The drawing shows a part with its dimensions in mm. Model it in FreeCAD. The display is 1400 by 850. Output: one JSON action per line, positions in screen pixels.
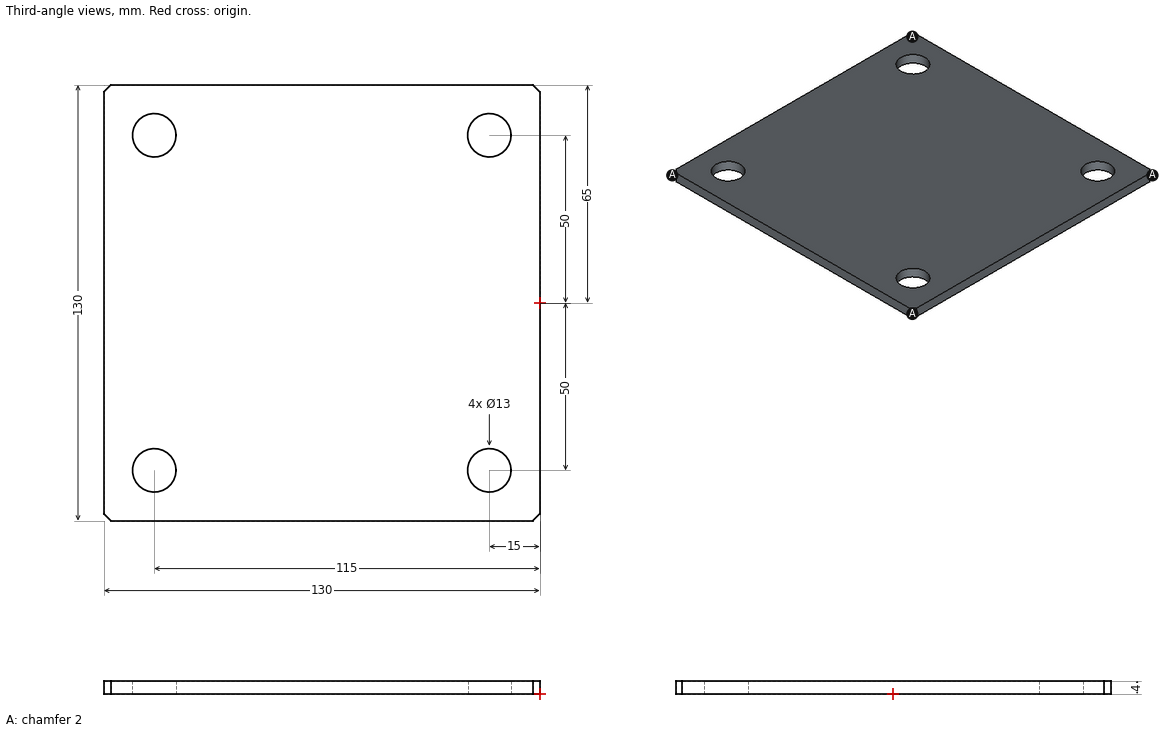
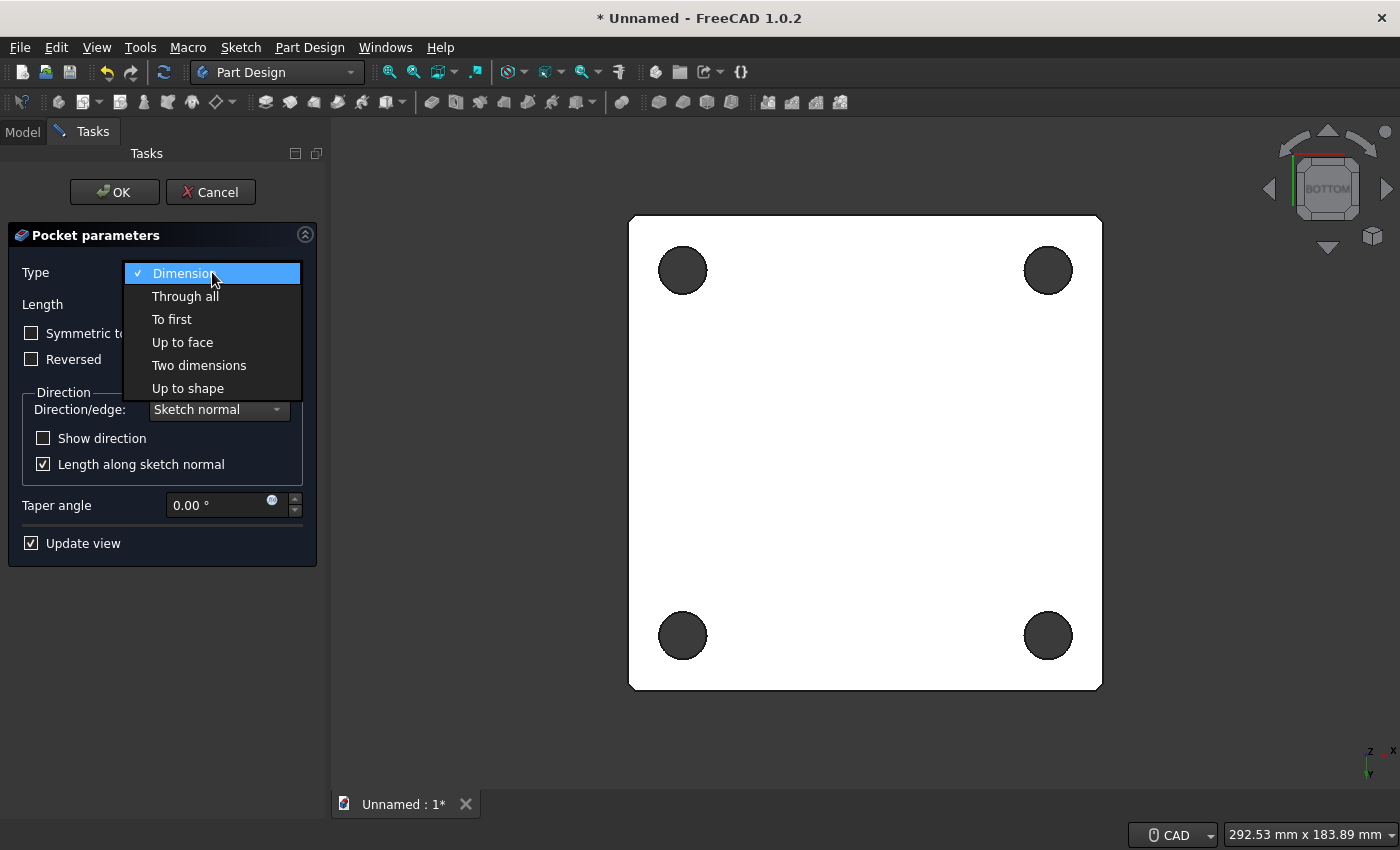
{"action": "left_click", "coordinate": [212, 296]}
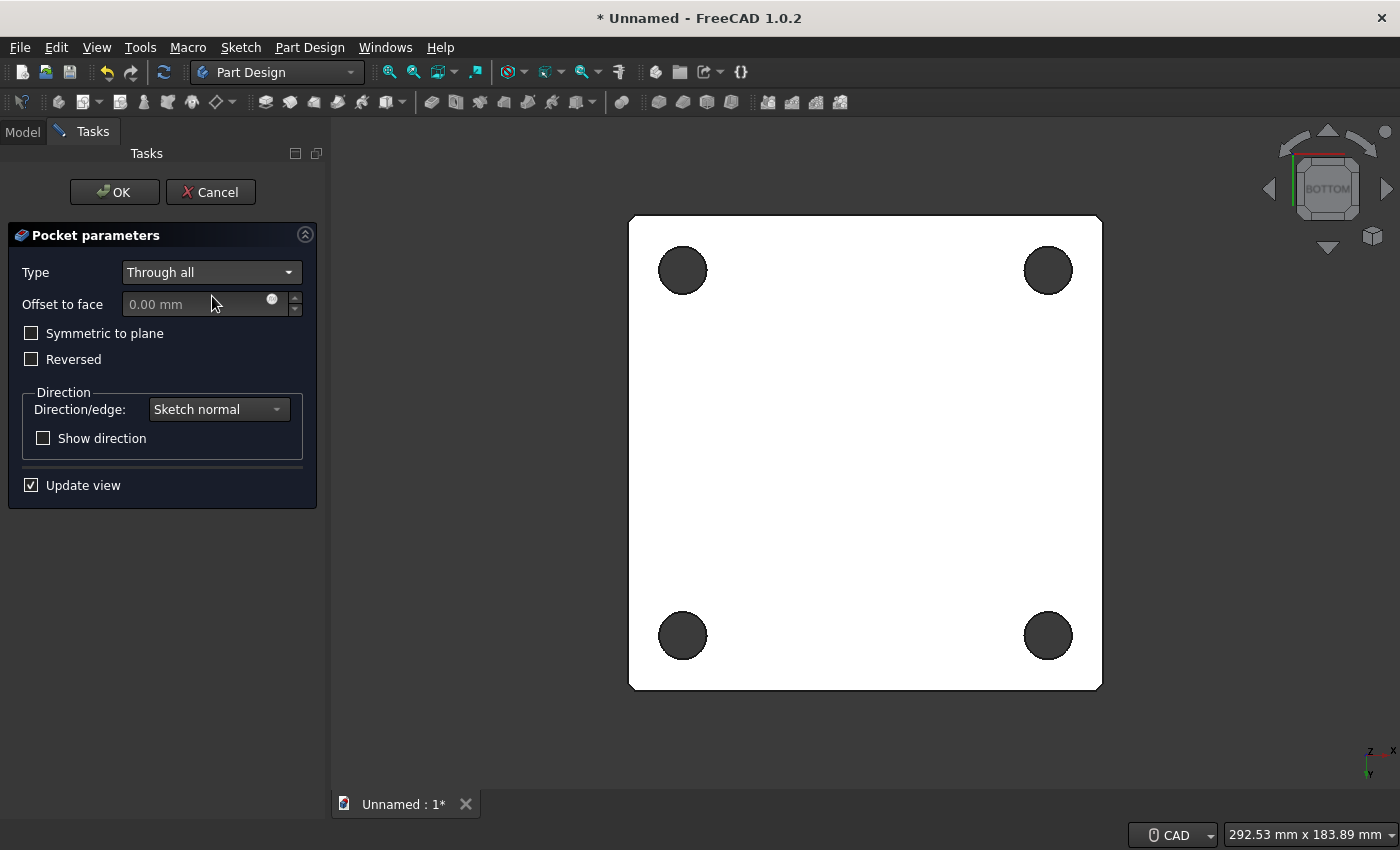
{"action": "left_click", "coordinate": [115, 192]}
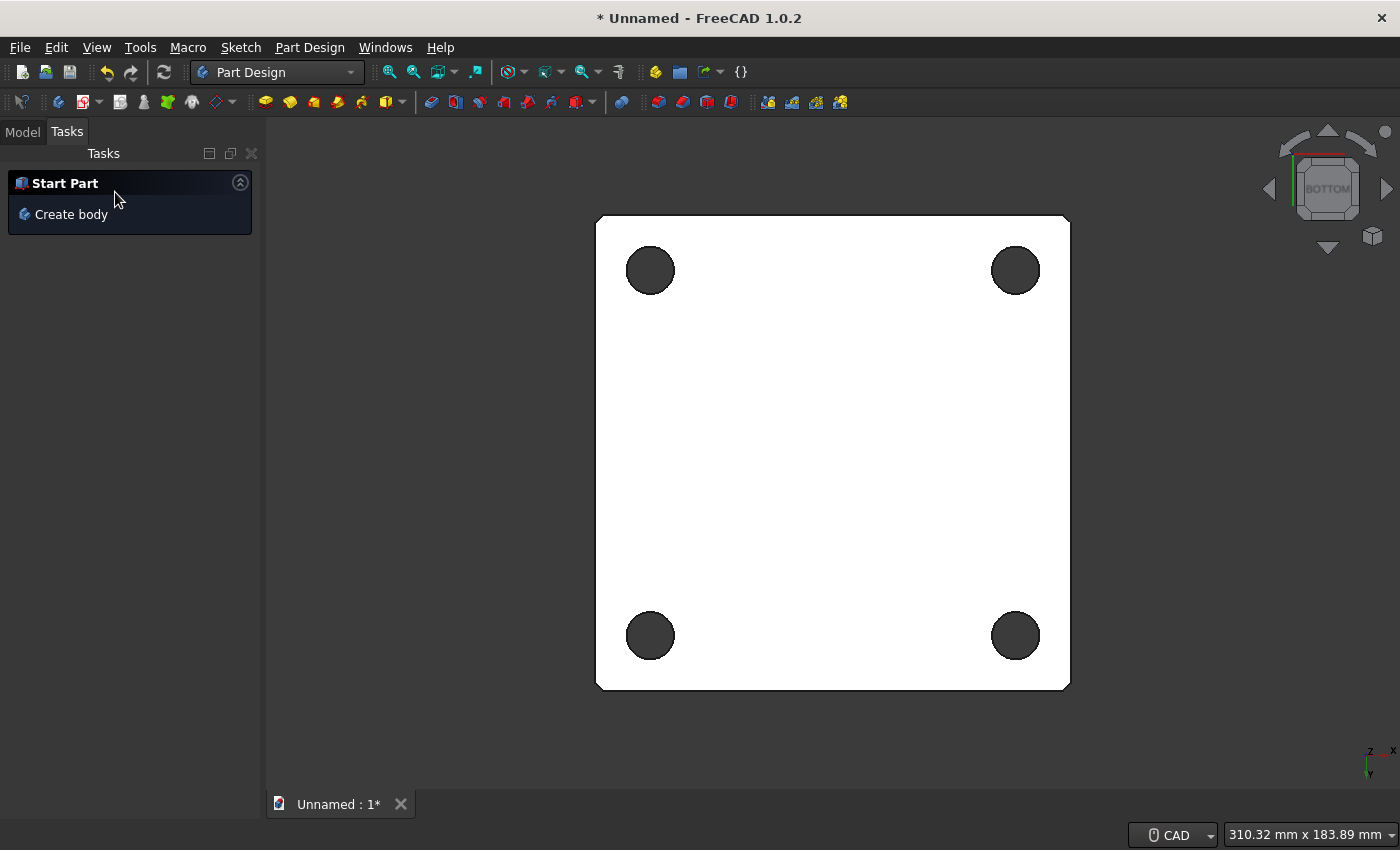
{"action": "key", "text": "0"}